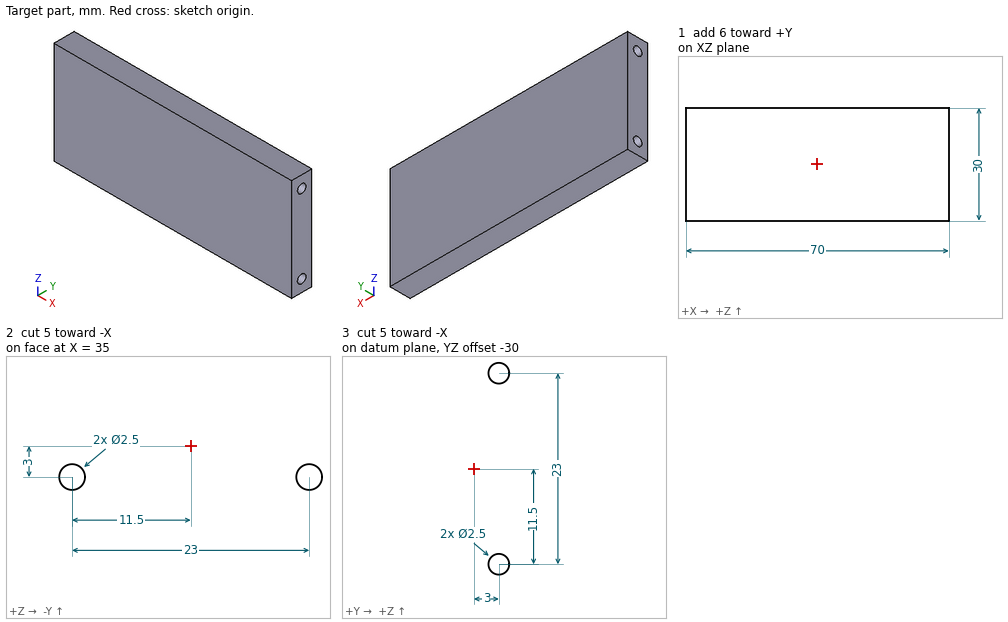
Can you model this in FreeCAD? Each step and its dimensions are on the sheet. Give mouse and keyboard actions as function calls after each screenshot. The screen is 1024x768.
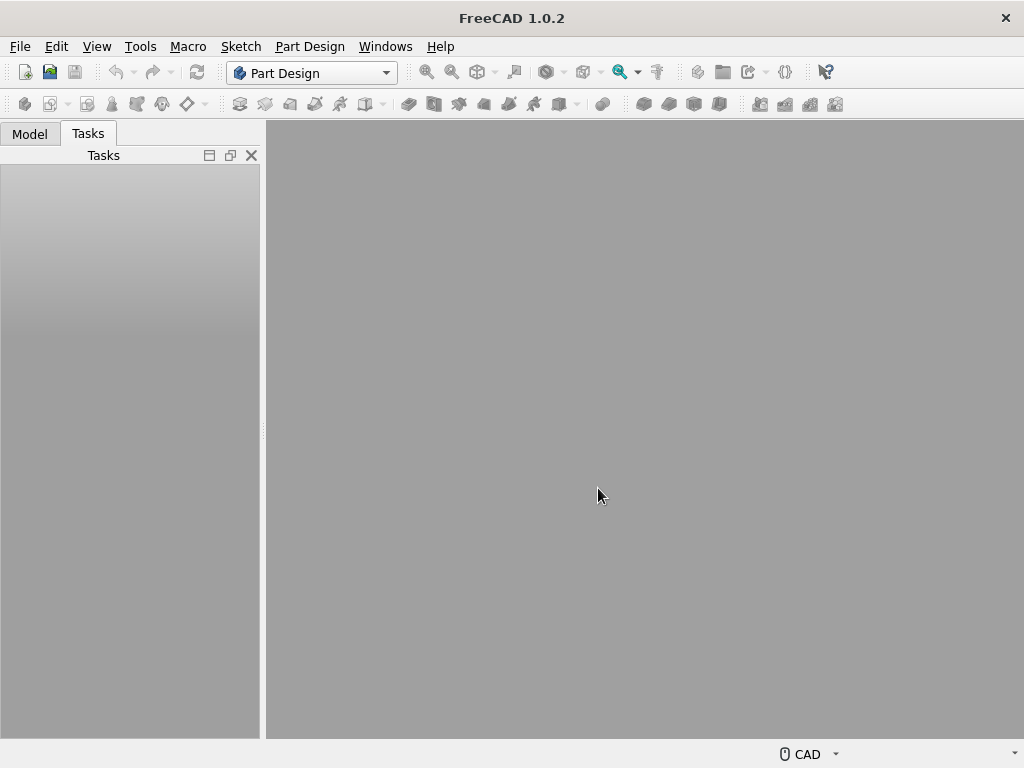
click(25, 72)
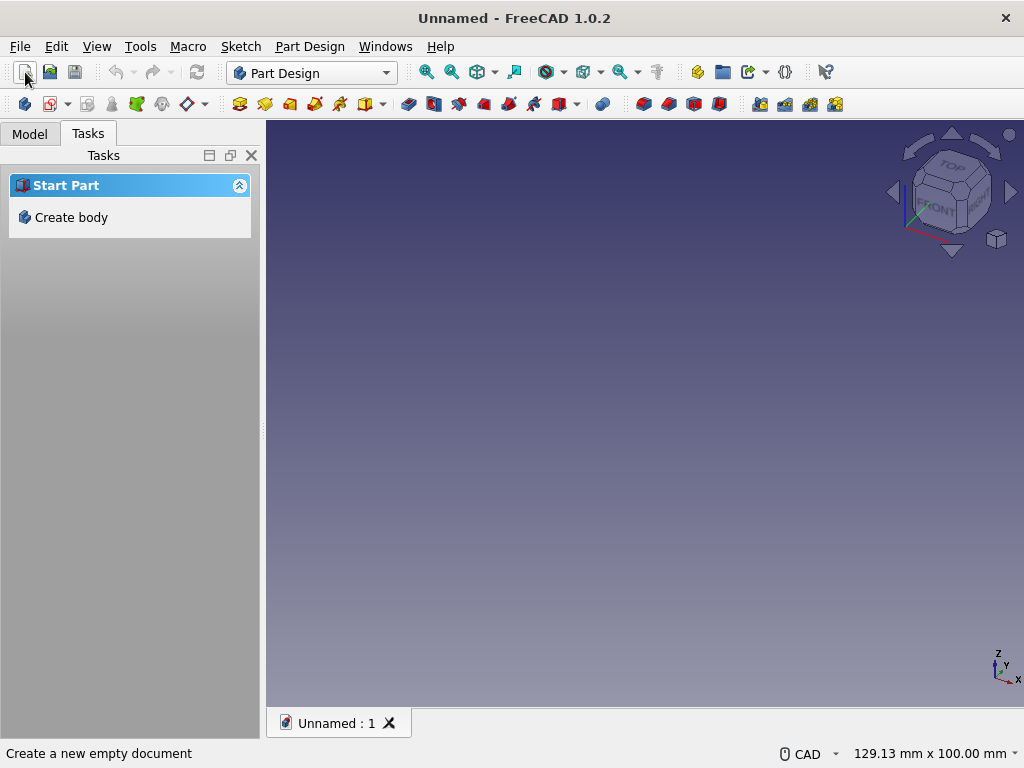
click(50, 104)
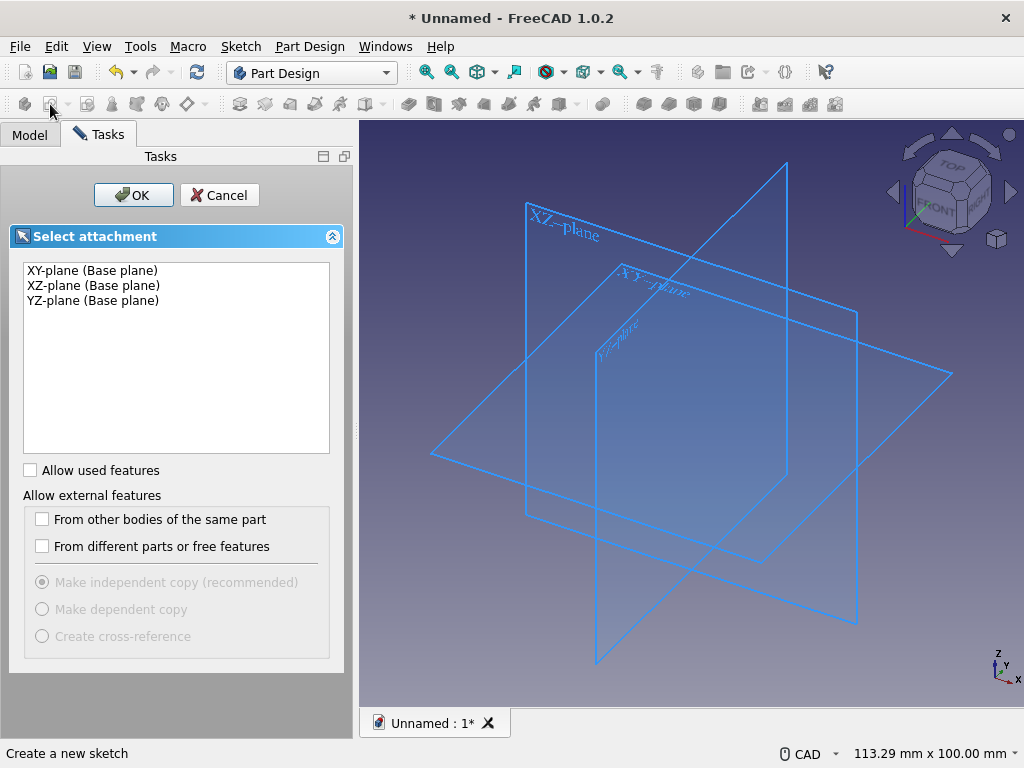
click(84, 286)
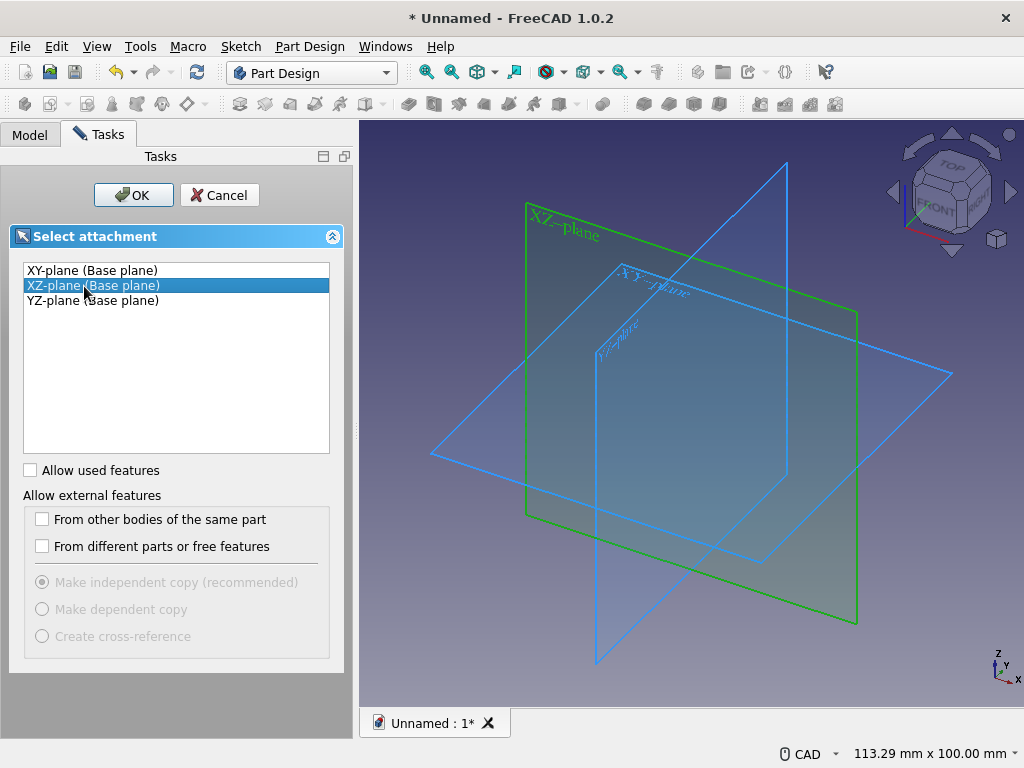
click(134, 195)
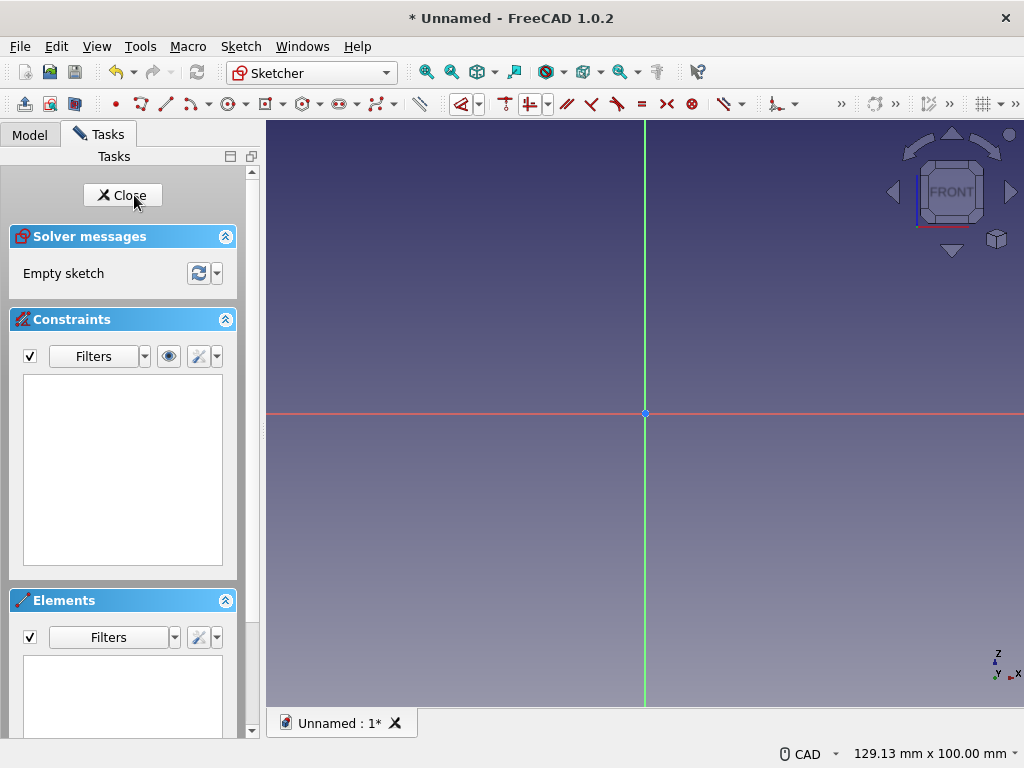
scroll(294, 413, down, 1)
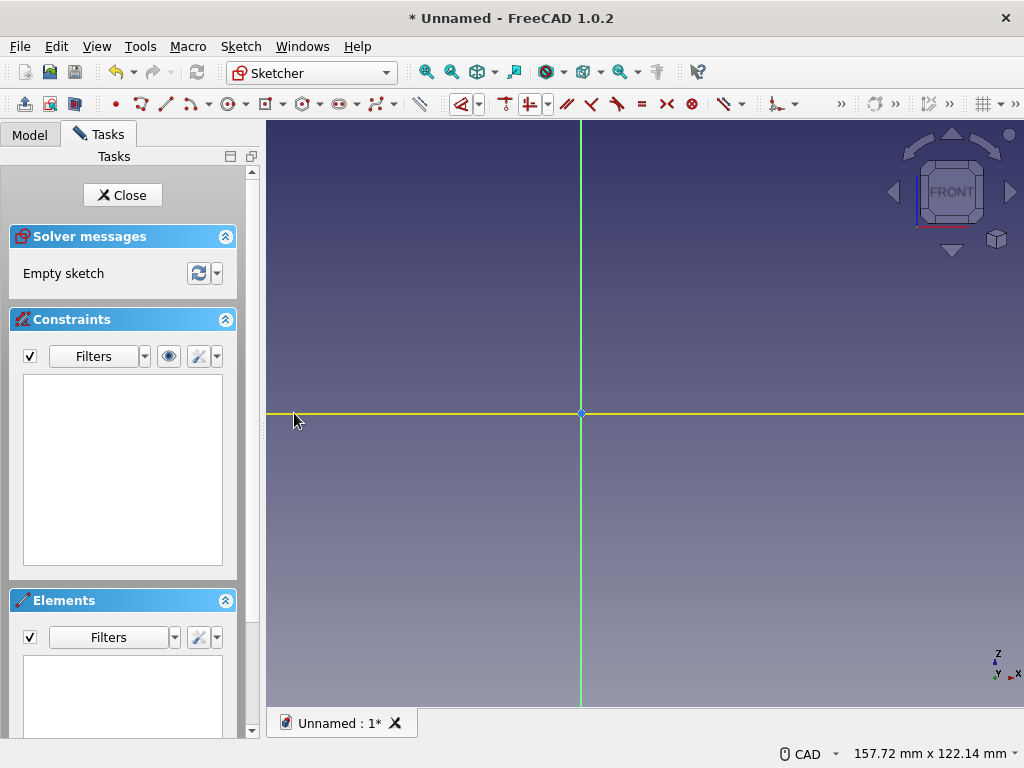
click(264, 104)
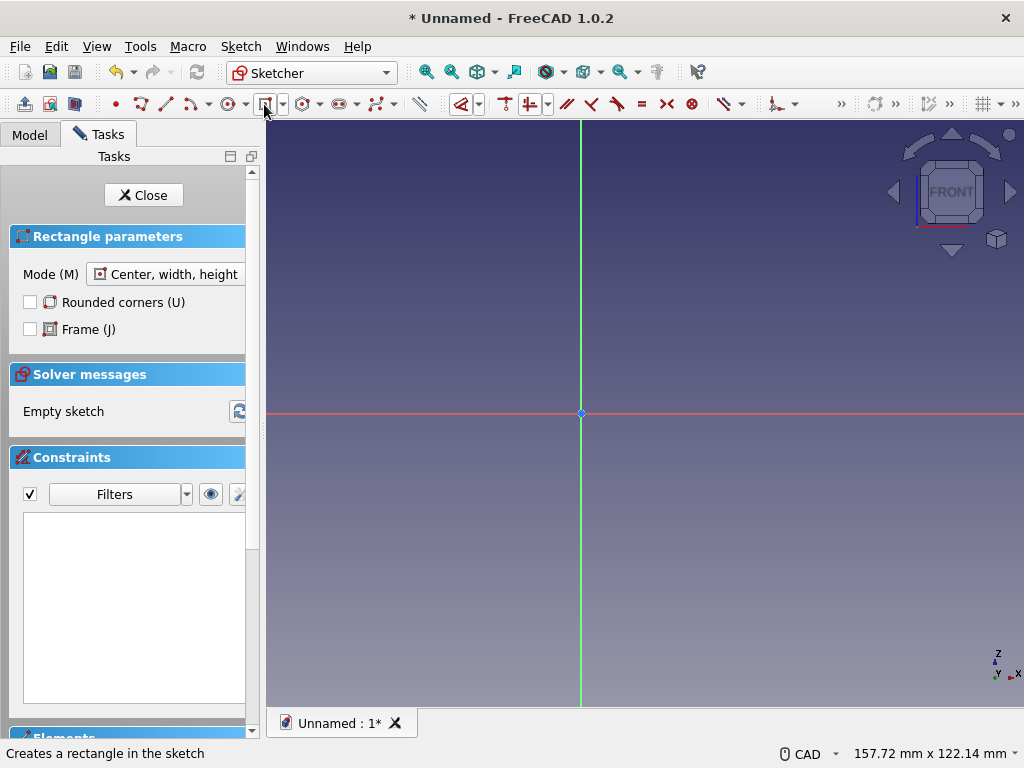
click(581, 414)
click(750, 341)
key(Escape)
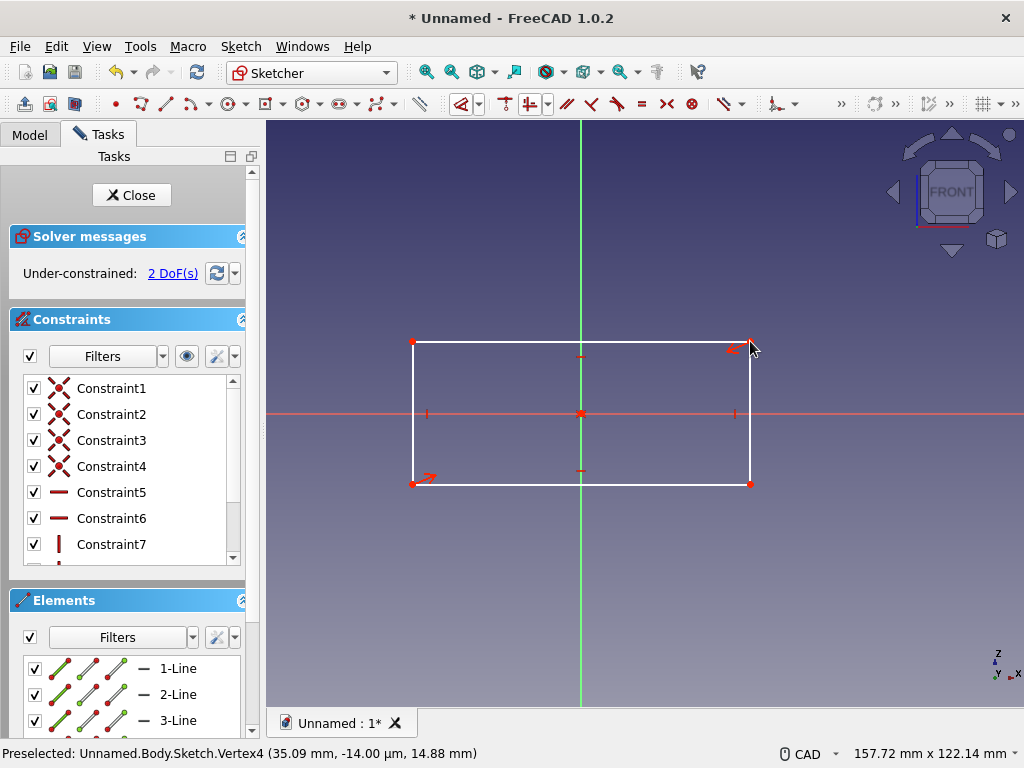
click(460, 104)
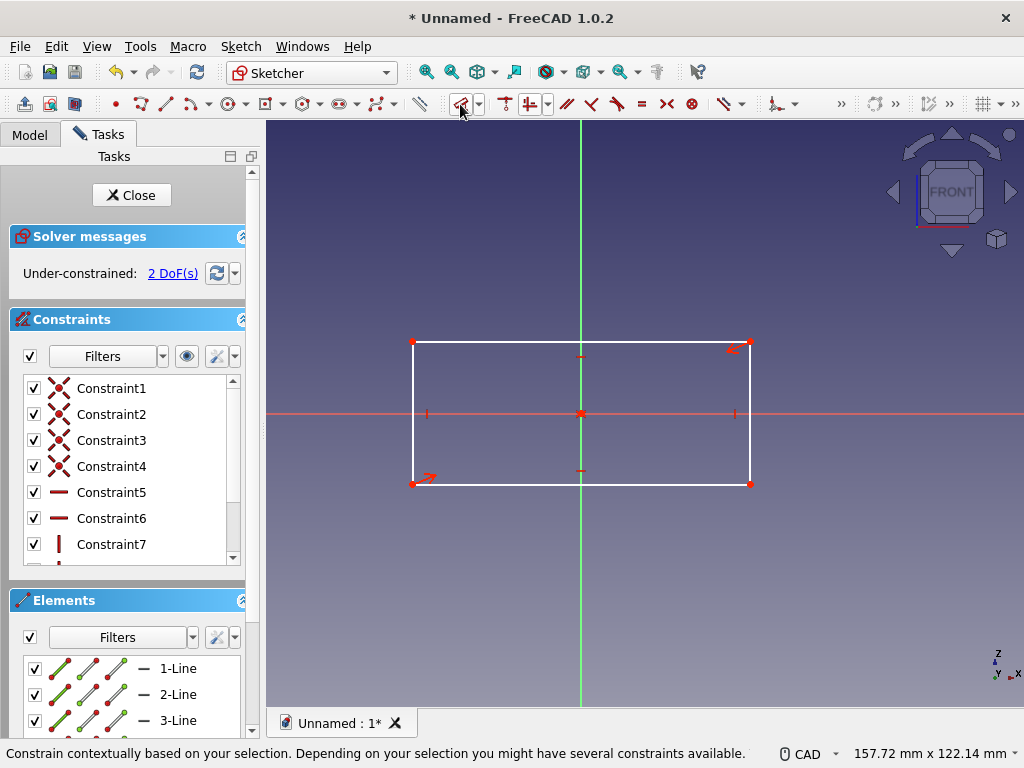
click(514, 485)
click(504, 519)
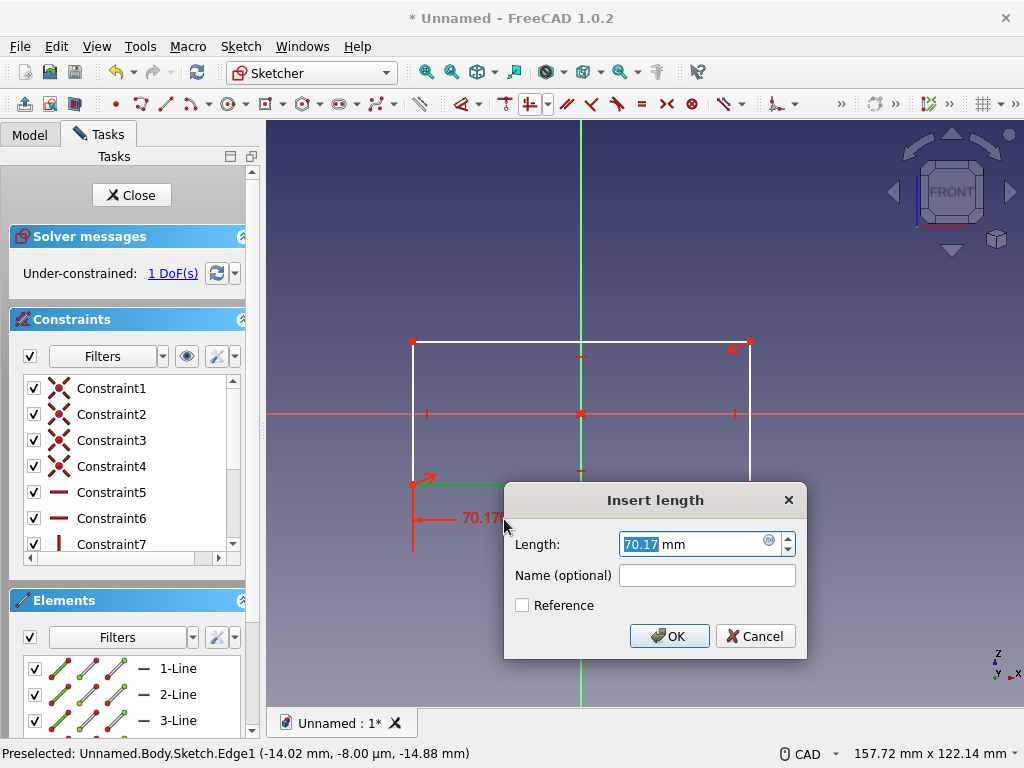
text(70)
key(Return)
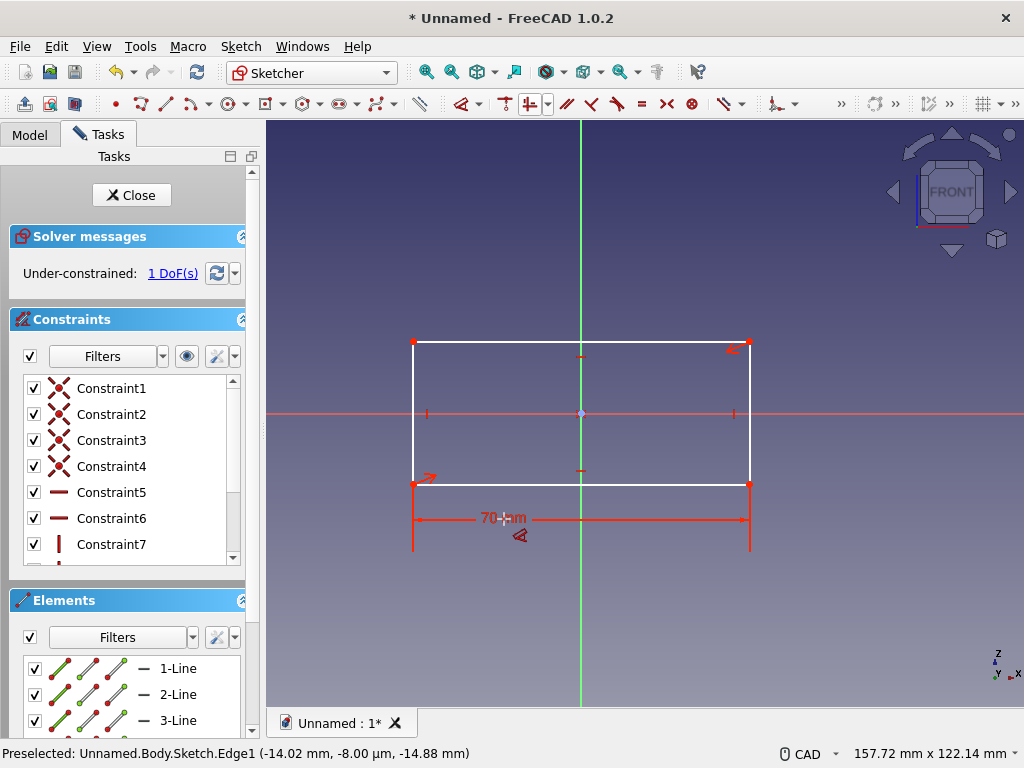
click(750, 442)
click(784, 381)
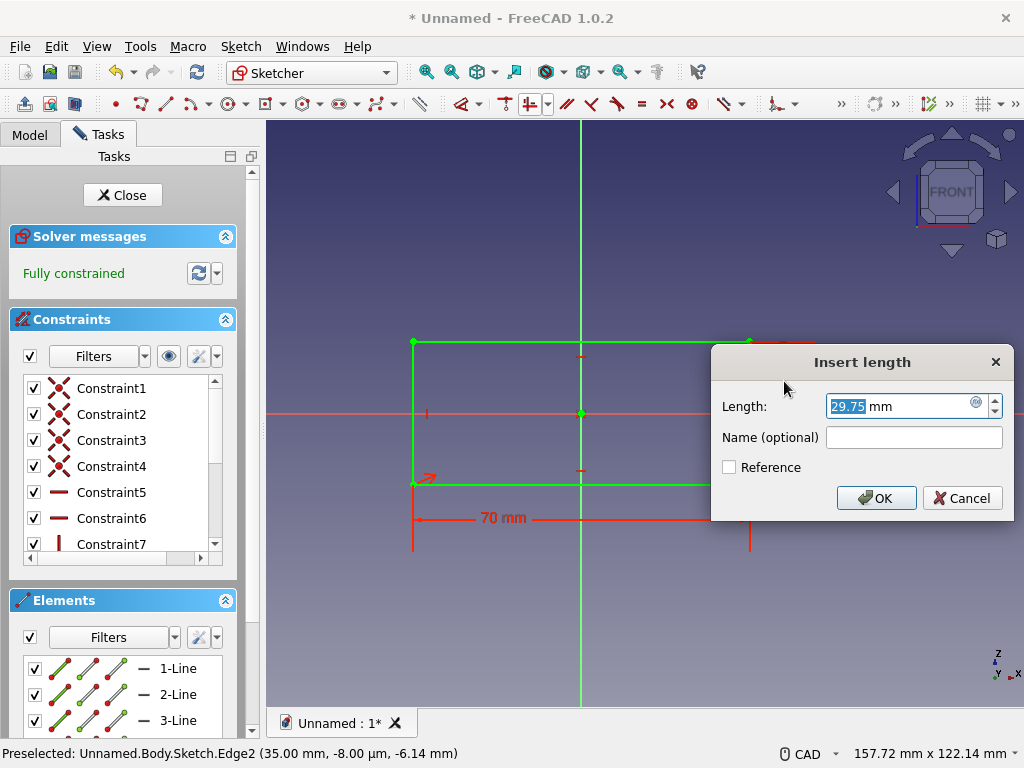
text(30)
key(Return)
key(Escape)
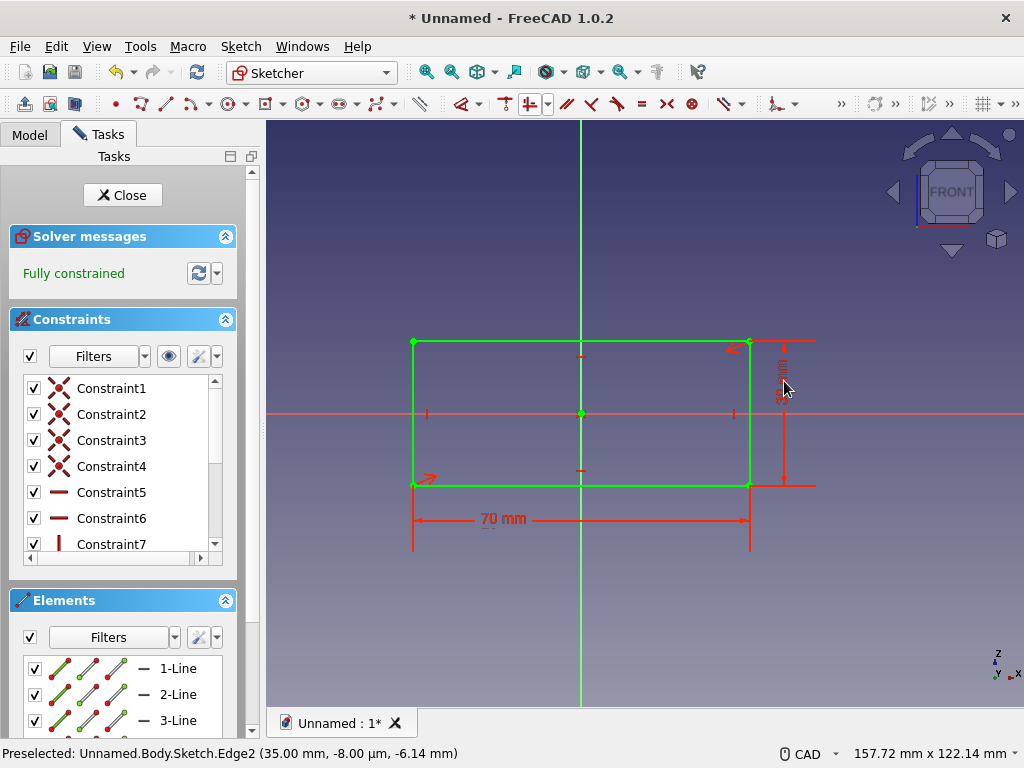
click(123, 195)